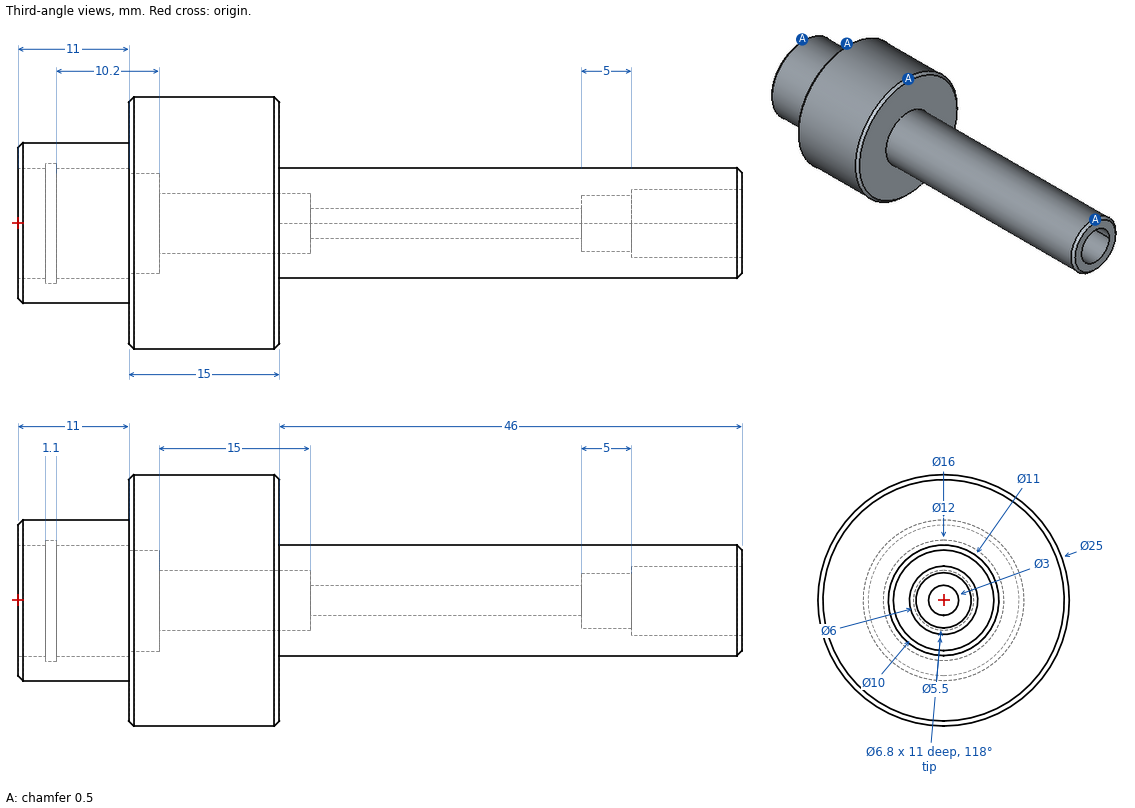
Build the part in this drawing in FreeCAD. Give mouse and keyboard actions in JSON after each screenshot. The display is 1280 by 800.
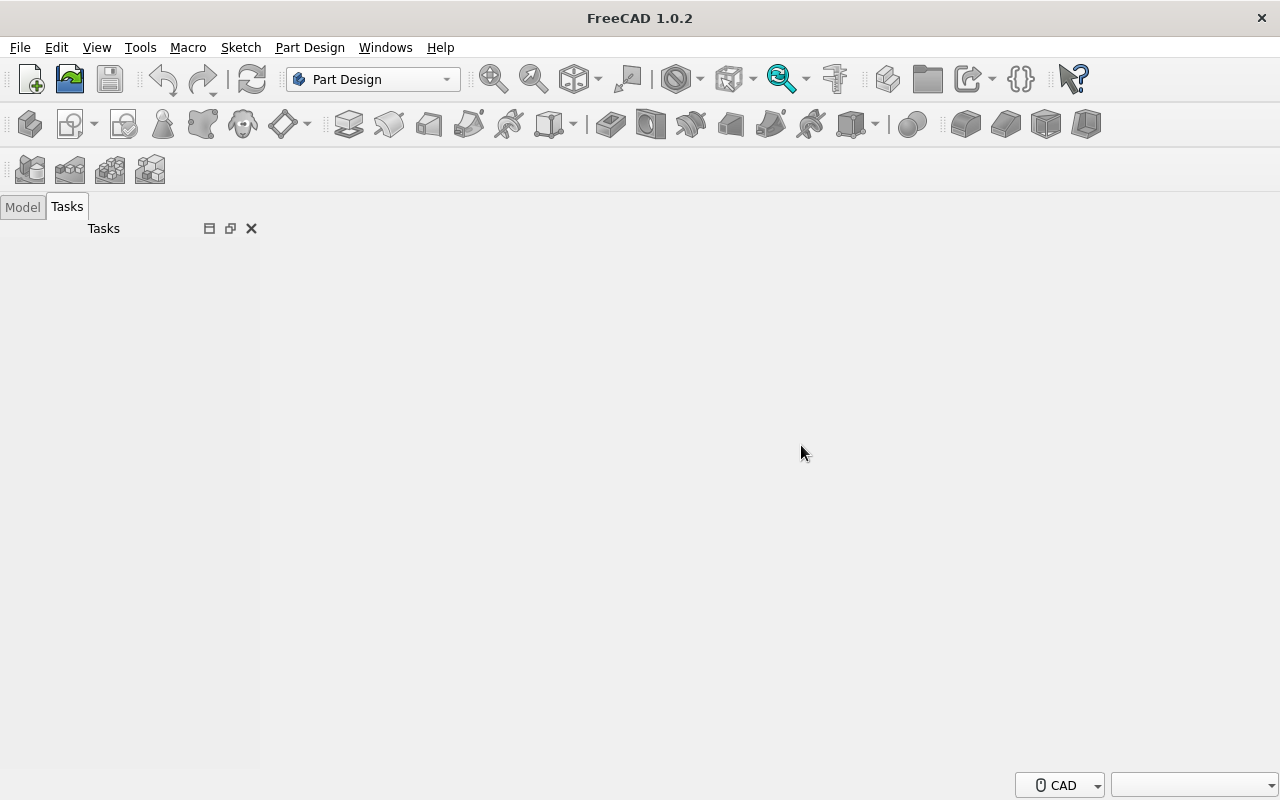
{"action": "left_click", "coordinate": [30, 80]}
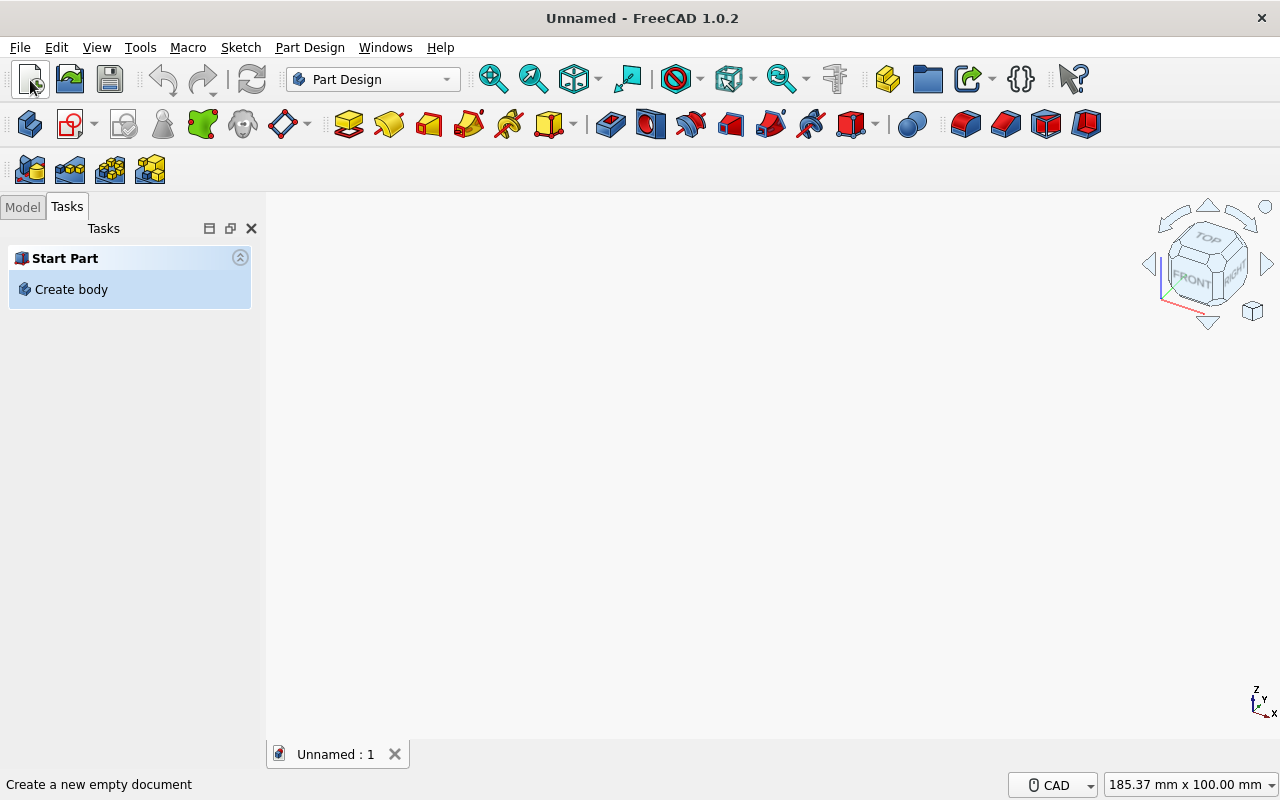
{"action": "left_click", "coordinate": [70, 124]}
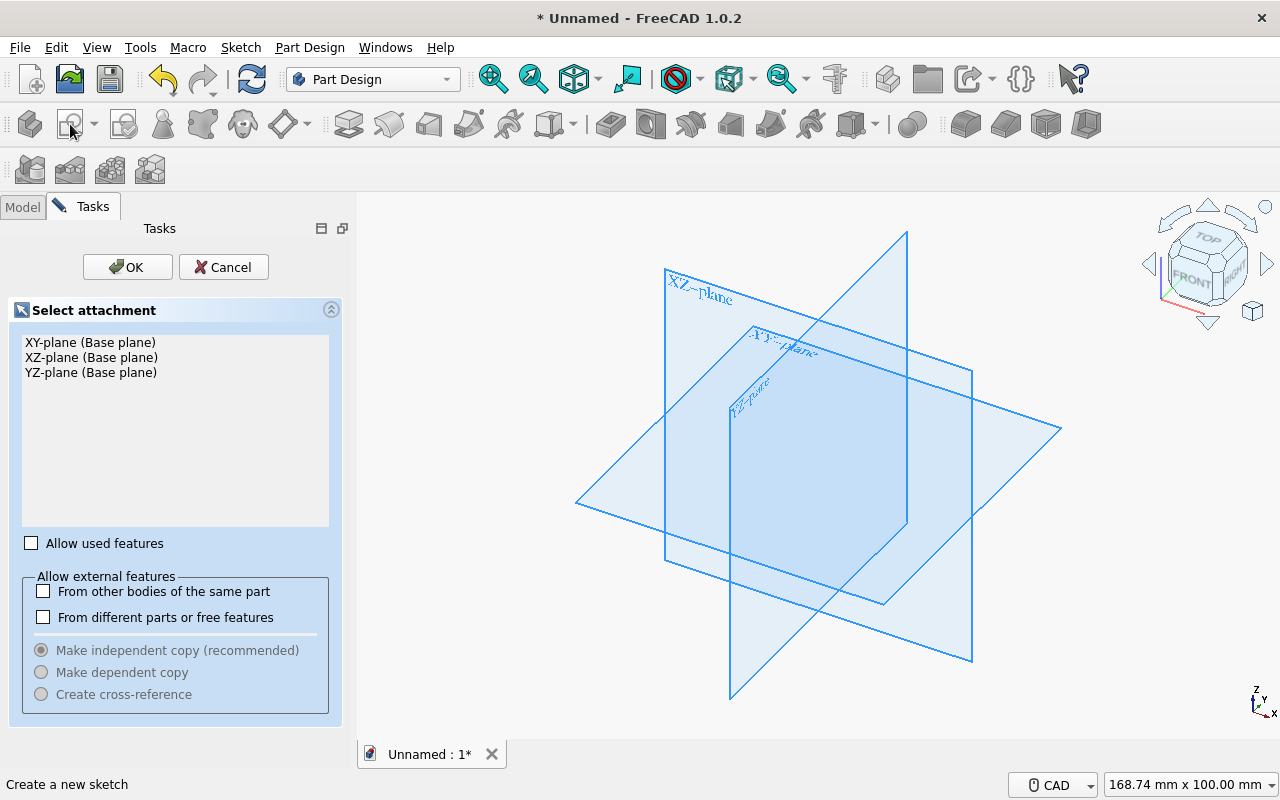
{"action": "left_click", "coordinate": [82, 372]}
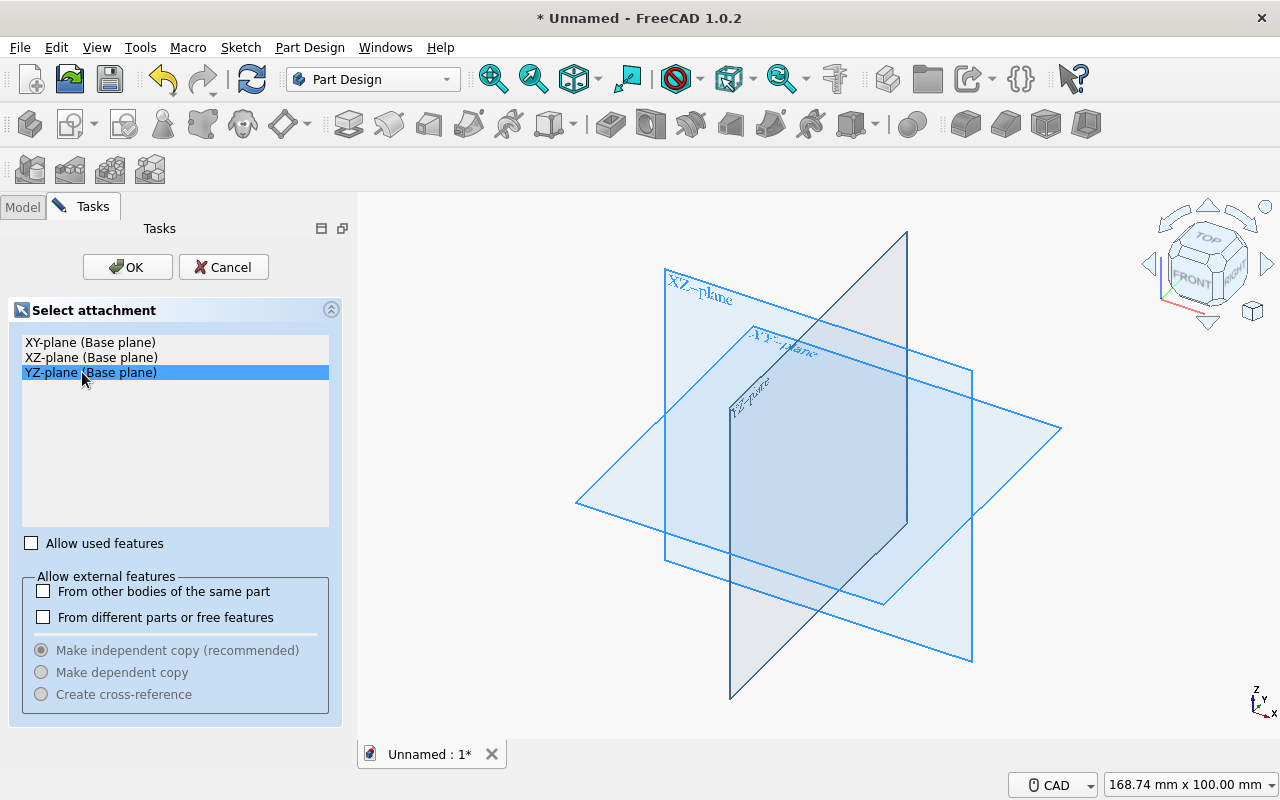
{"action": "left_click", "coordinate": [128, 267]}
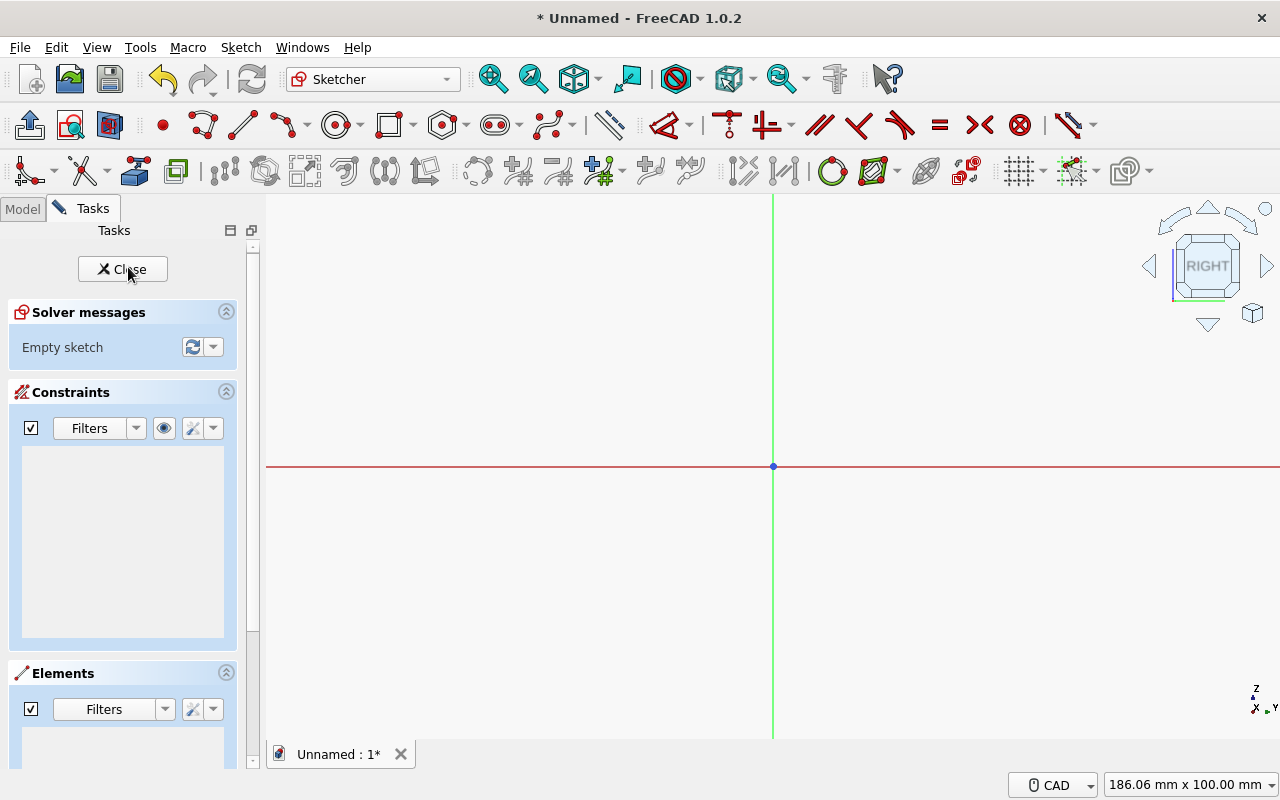
{"action": "scroll", "coordinate": [795, 466], "scroll_direction": "up", "scroll_amount": 7}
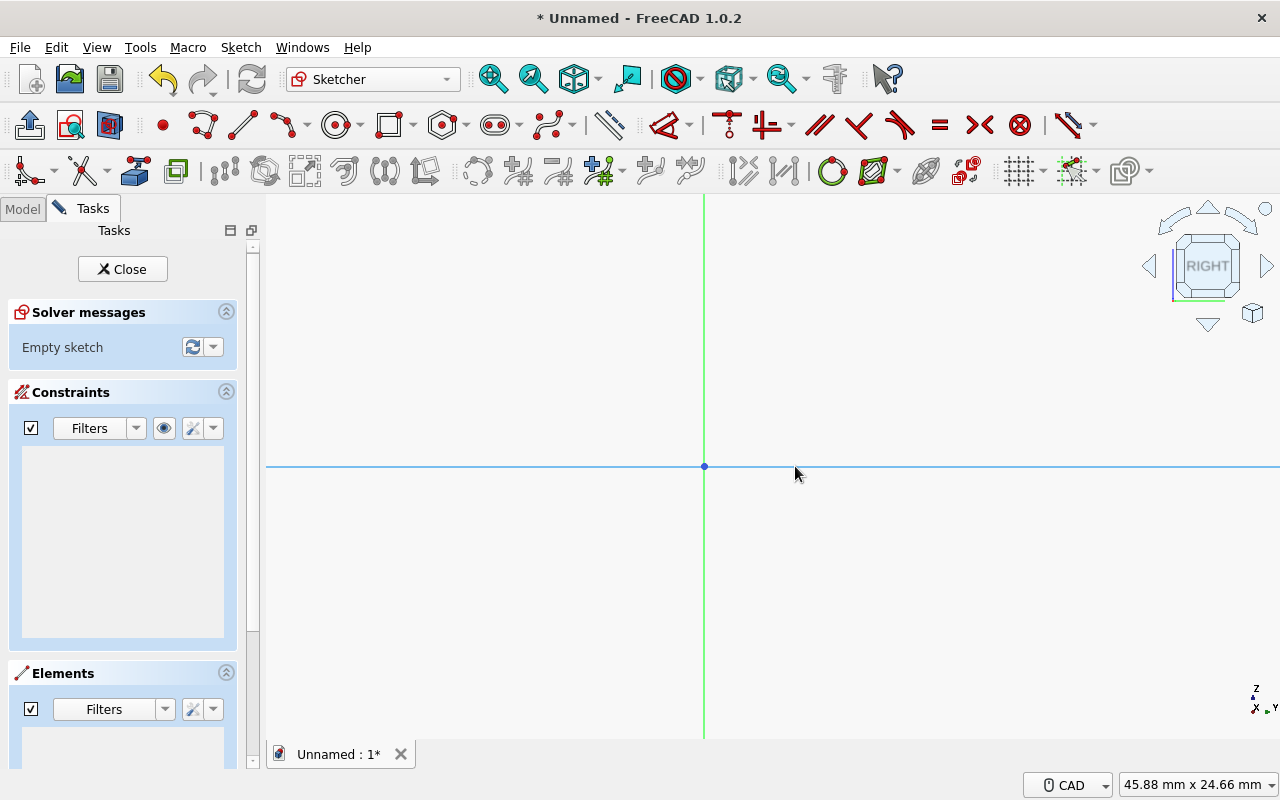
{"action": "left_click", "coordinate": [336, 126]}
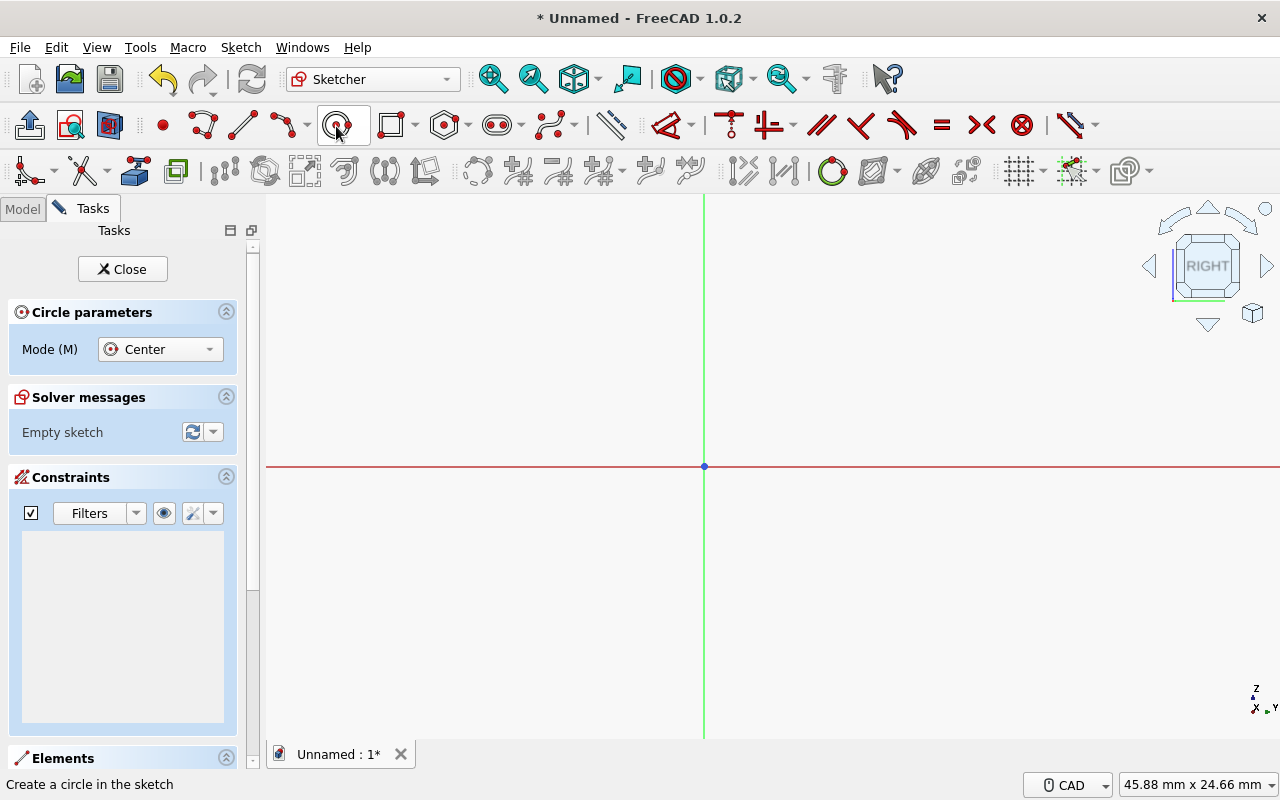
{"action": "left_click", "coordinate": [704, 466]}
{"action": "mouse_move", "coordinate": [829, 341]}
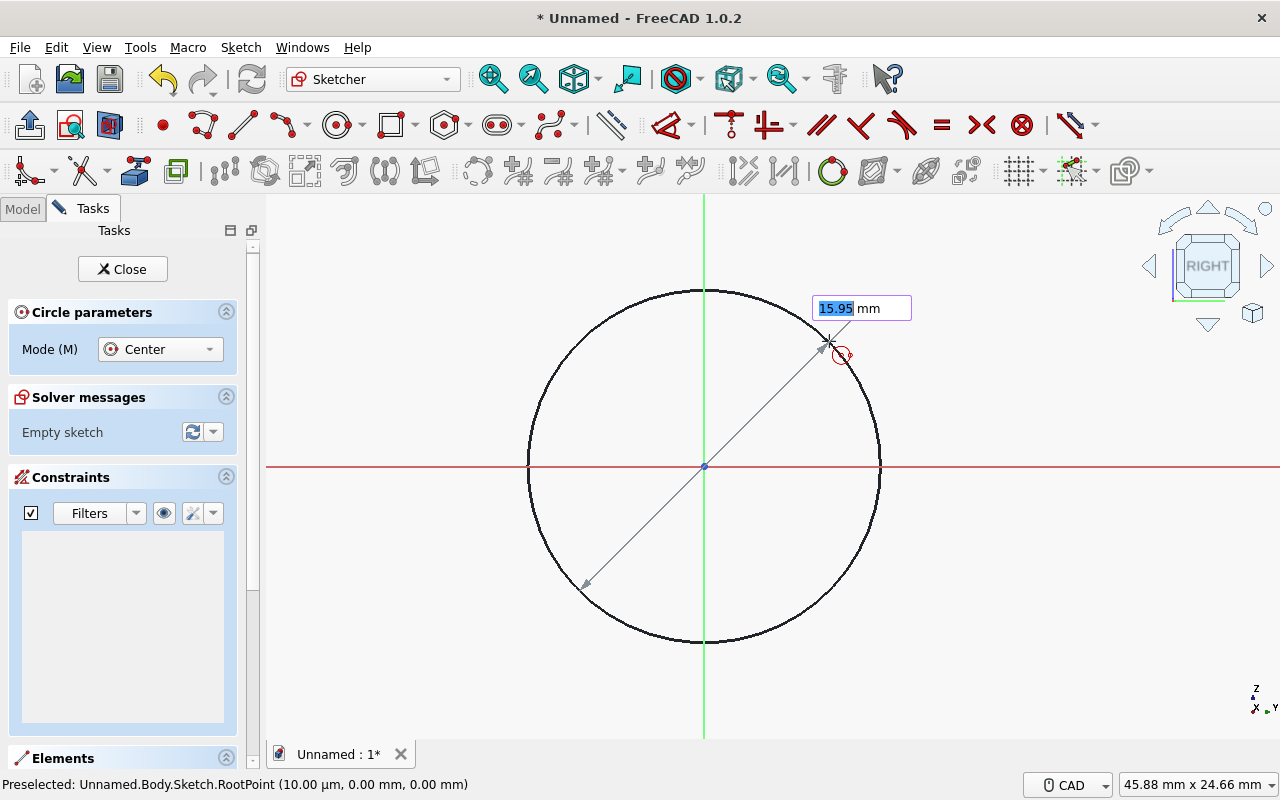
{"action": "type", "text": "16"}
{"action": "key", "text": "Return"}
{"action": "key", "text": "Escape"}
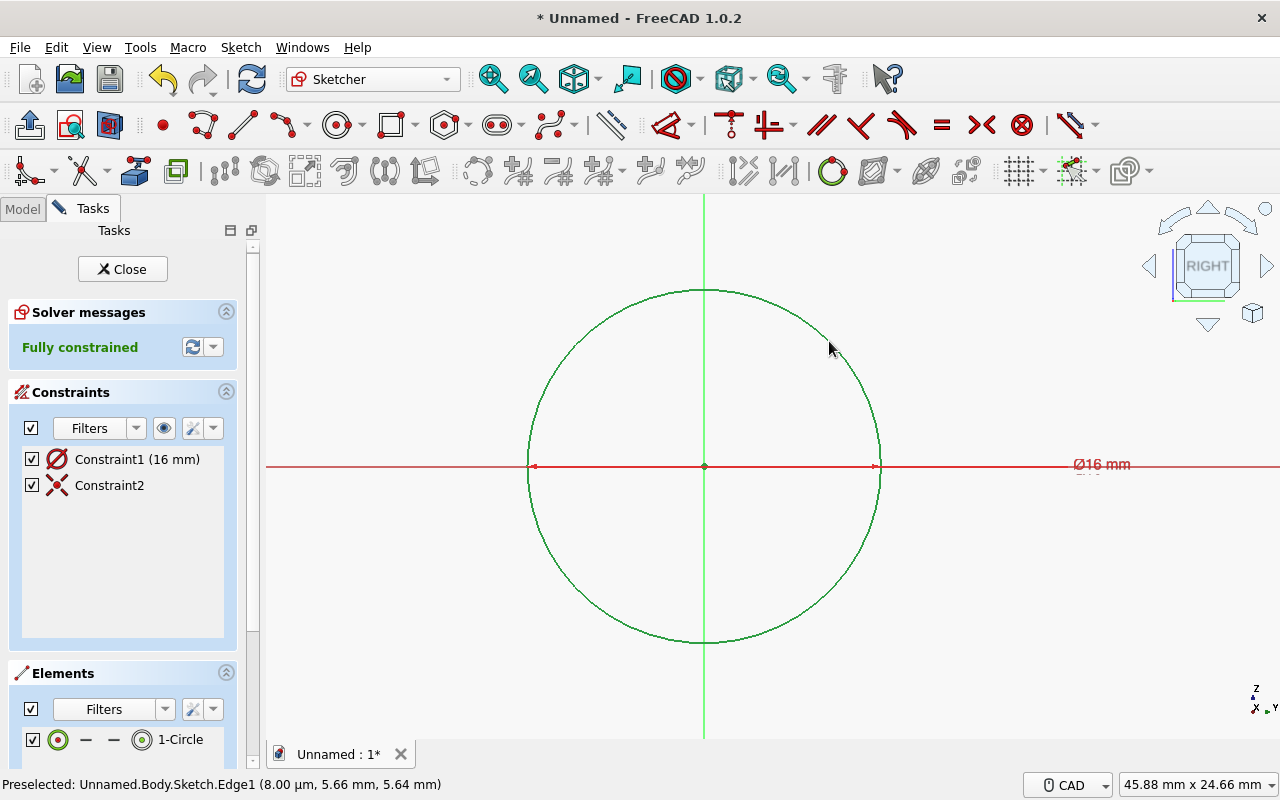
{"action": "left_click", "coordinate": [123, 269]}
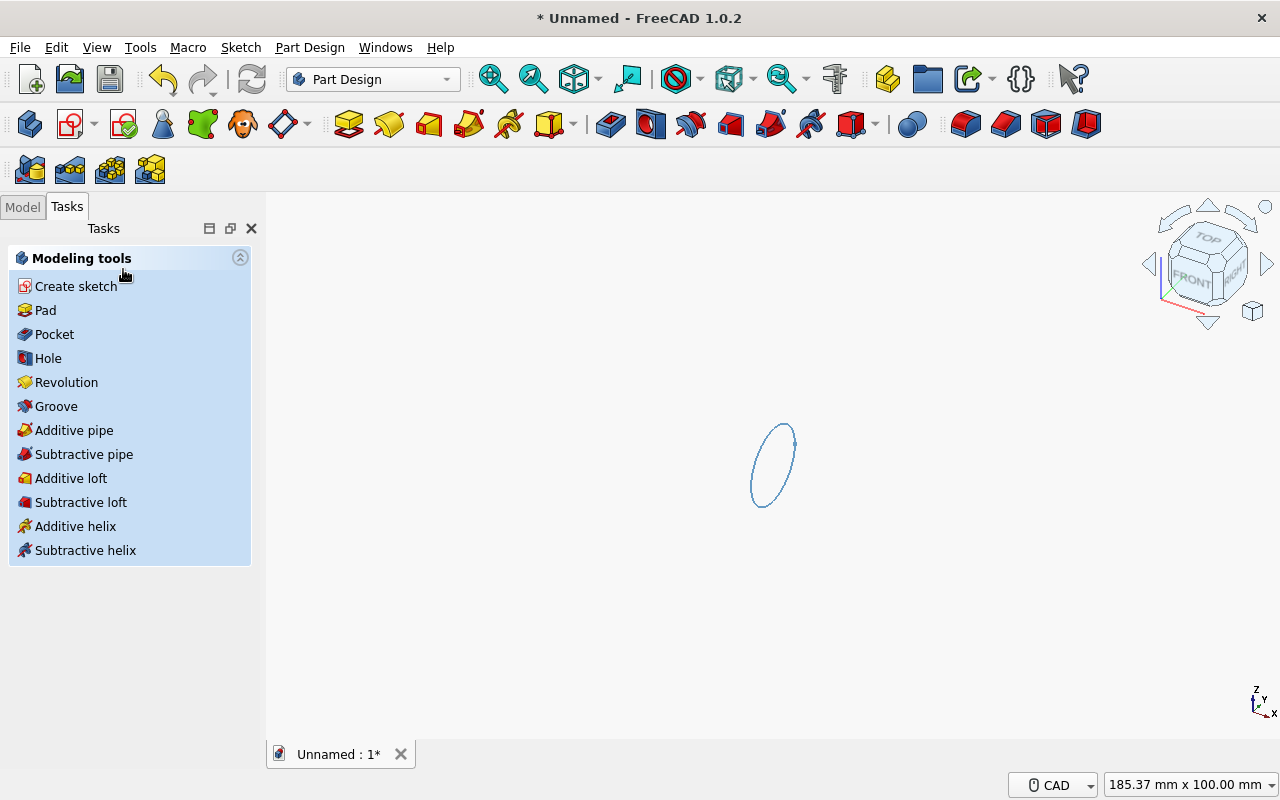
{"action": "left_click", "coordinate": [350, 124]}